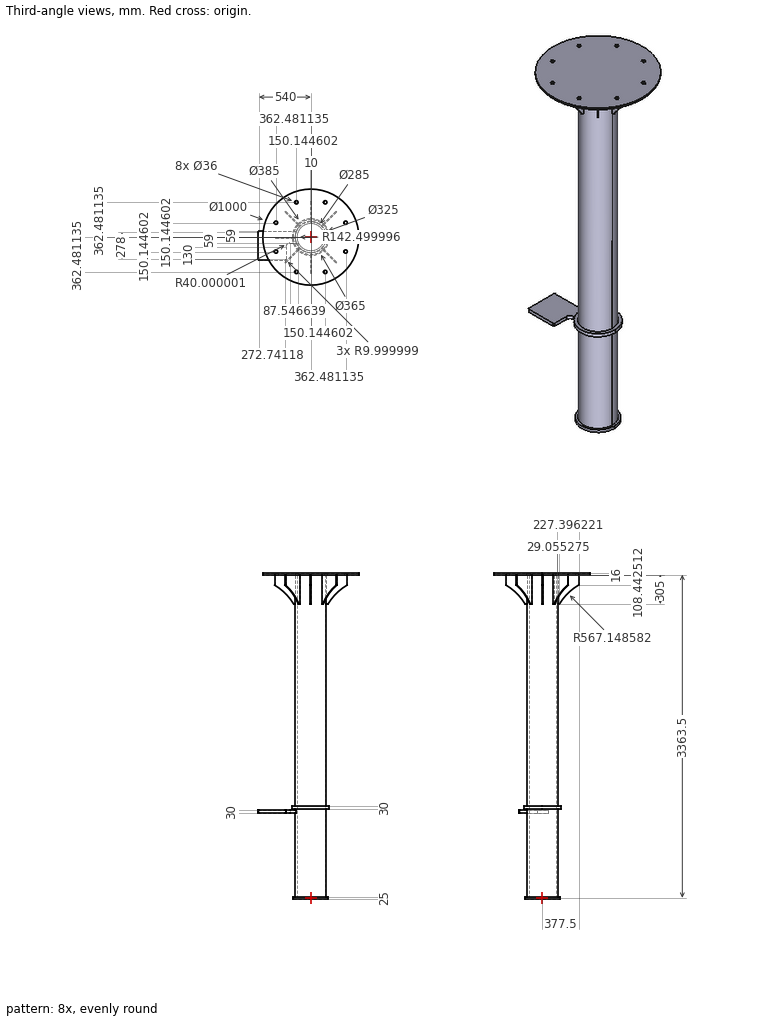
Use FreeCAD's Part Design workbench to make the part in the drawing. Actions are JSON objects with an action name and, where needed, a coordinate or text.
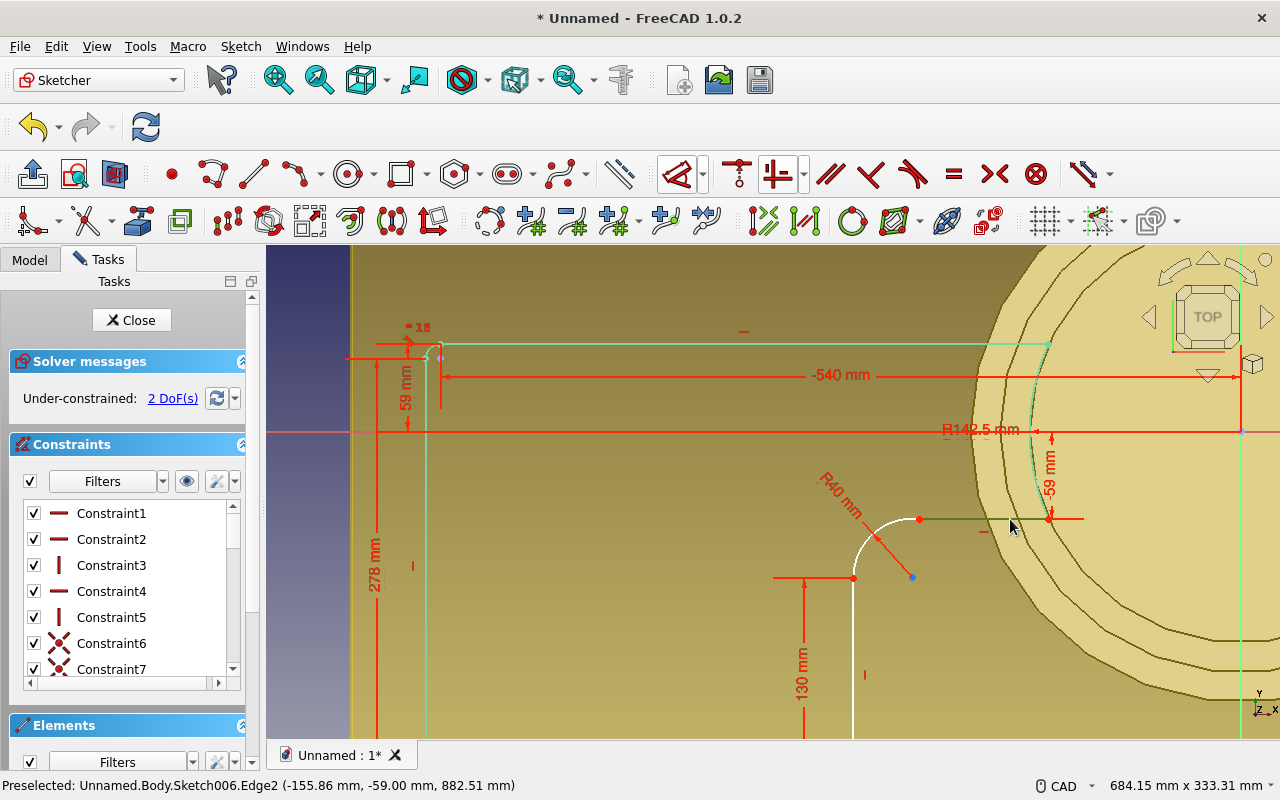
{"action": "key", "text": "l"}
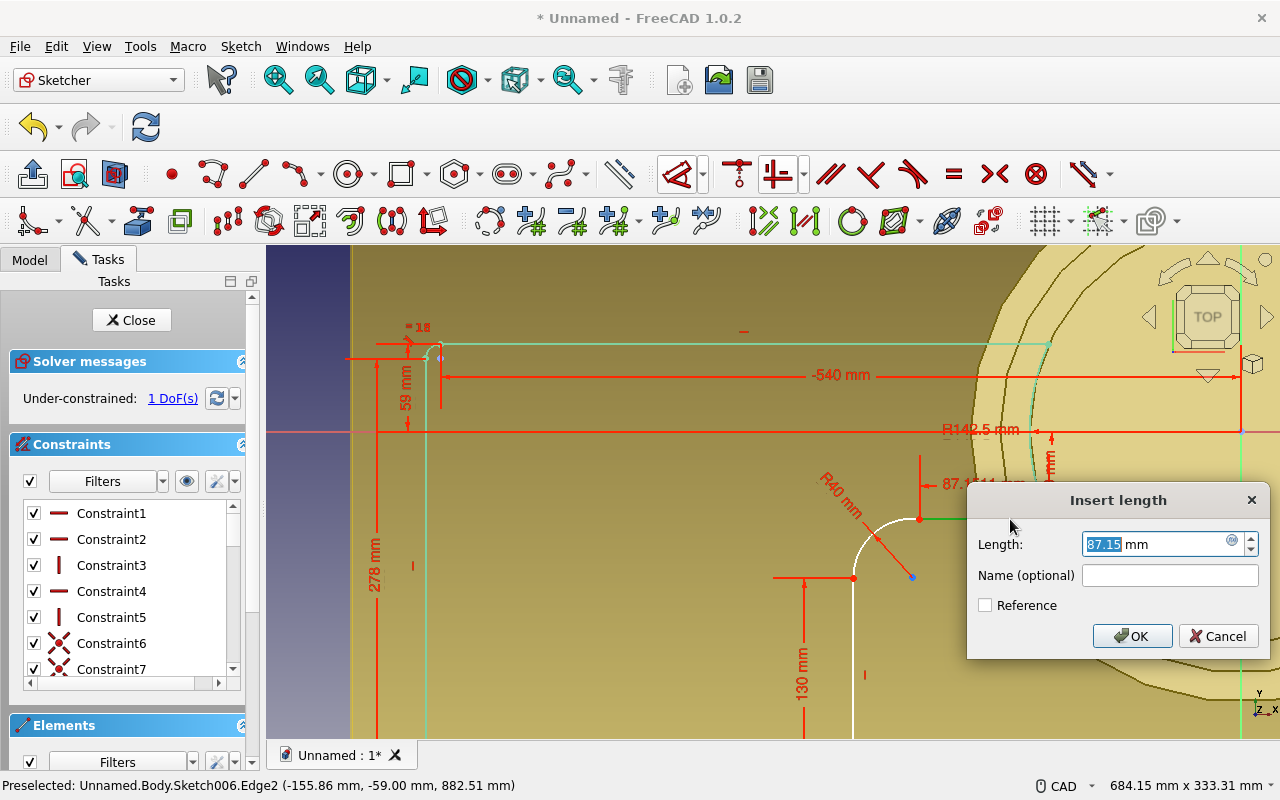
{"action": "type", "text": "87.546639"}
{"action": "key", "text": "Return"}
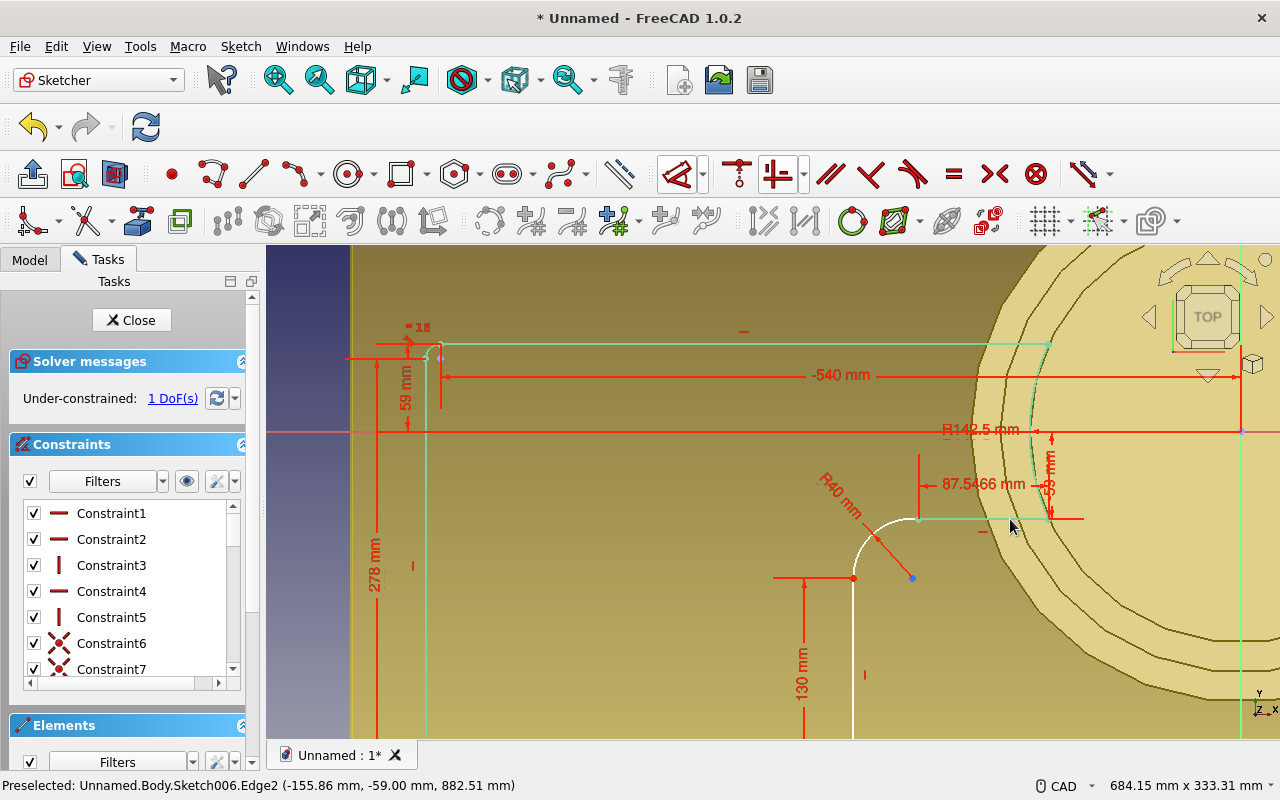
{"action": "scroll", "coordinate": [442, 344], "scroll_direction": "down", "scroll_amount": 2}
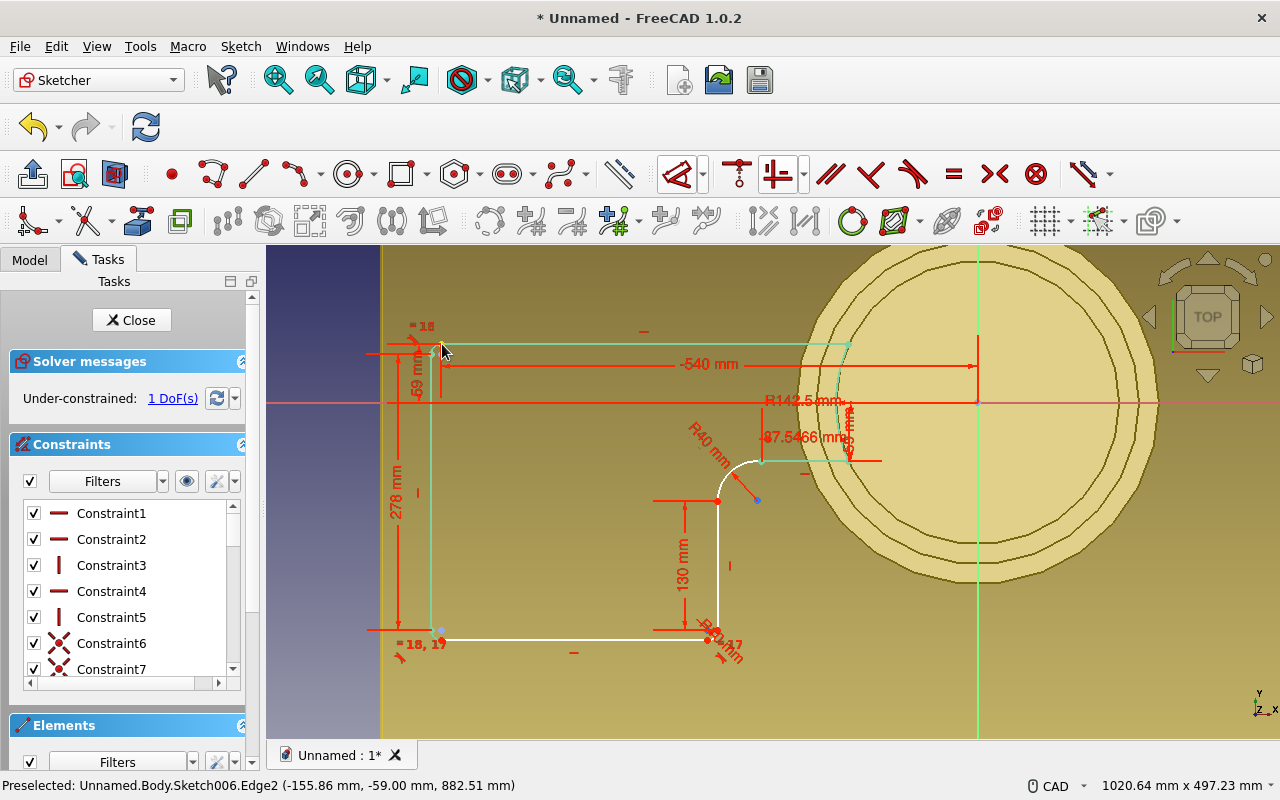
{"action": "left_click", "coordinate": [628, 640]}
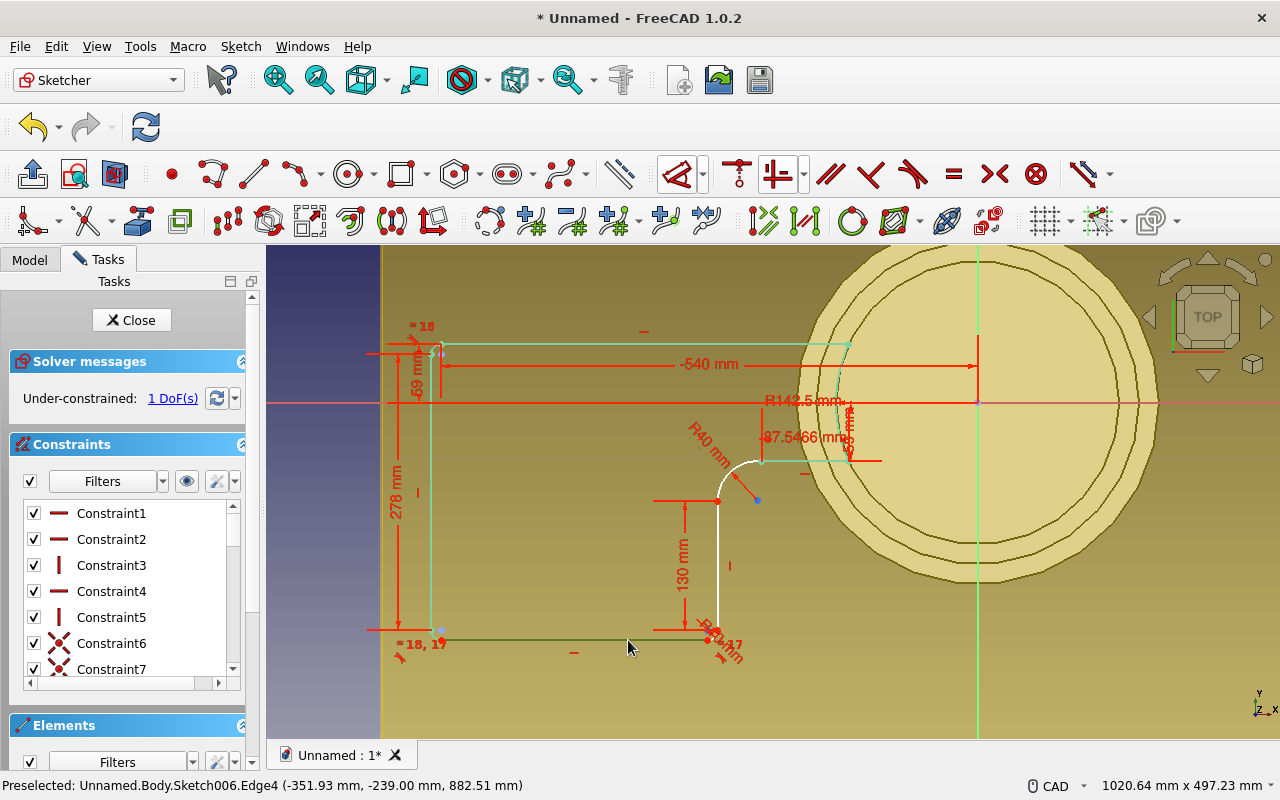
{"action": "left_click", "coordinate": [702, 174]}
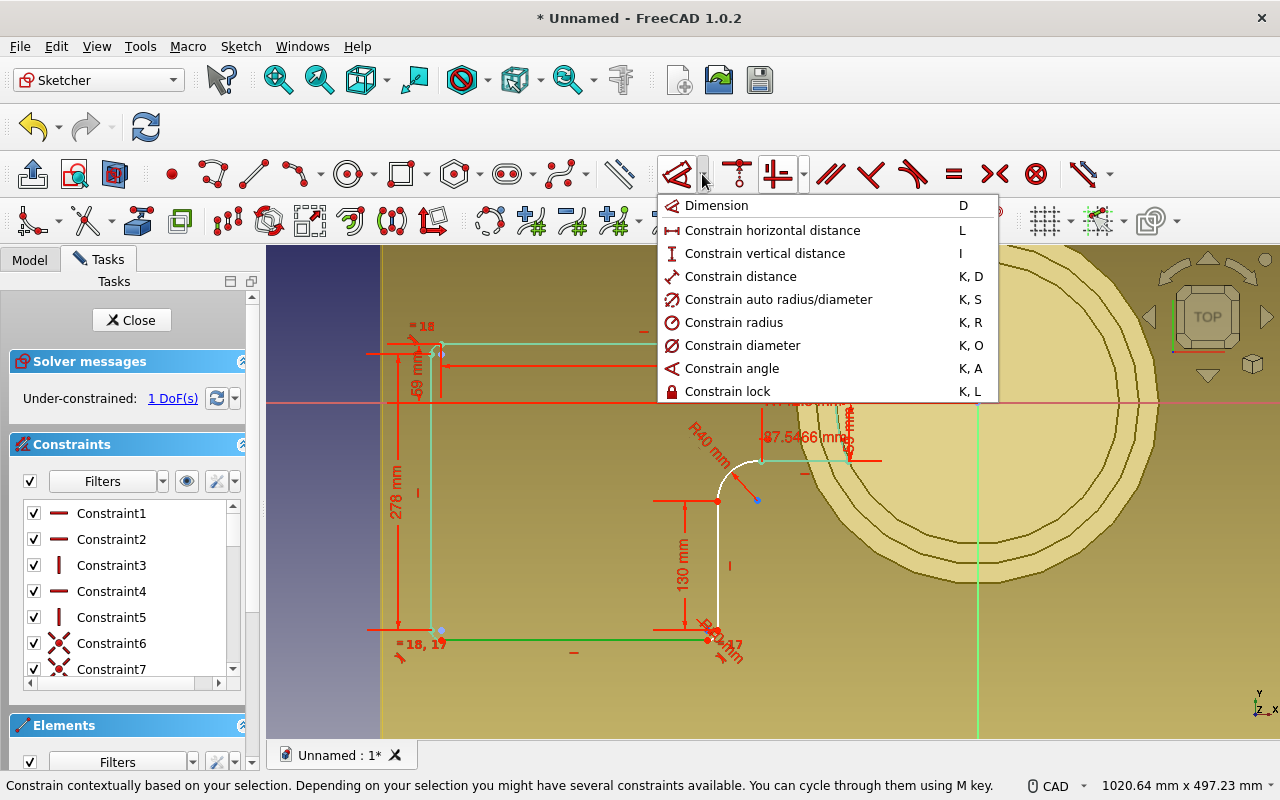
{"action": "left_click", "coordinate": [828, 230]}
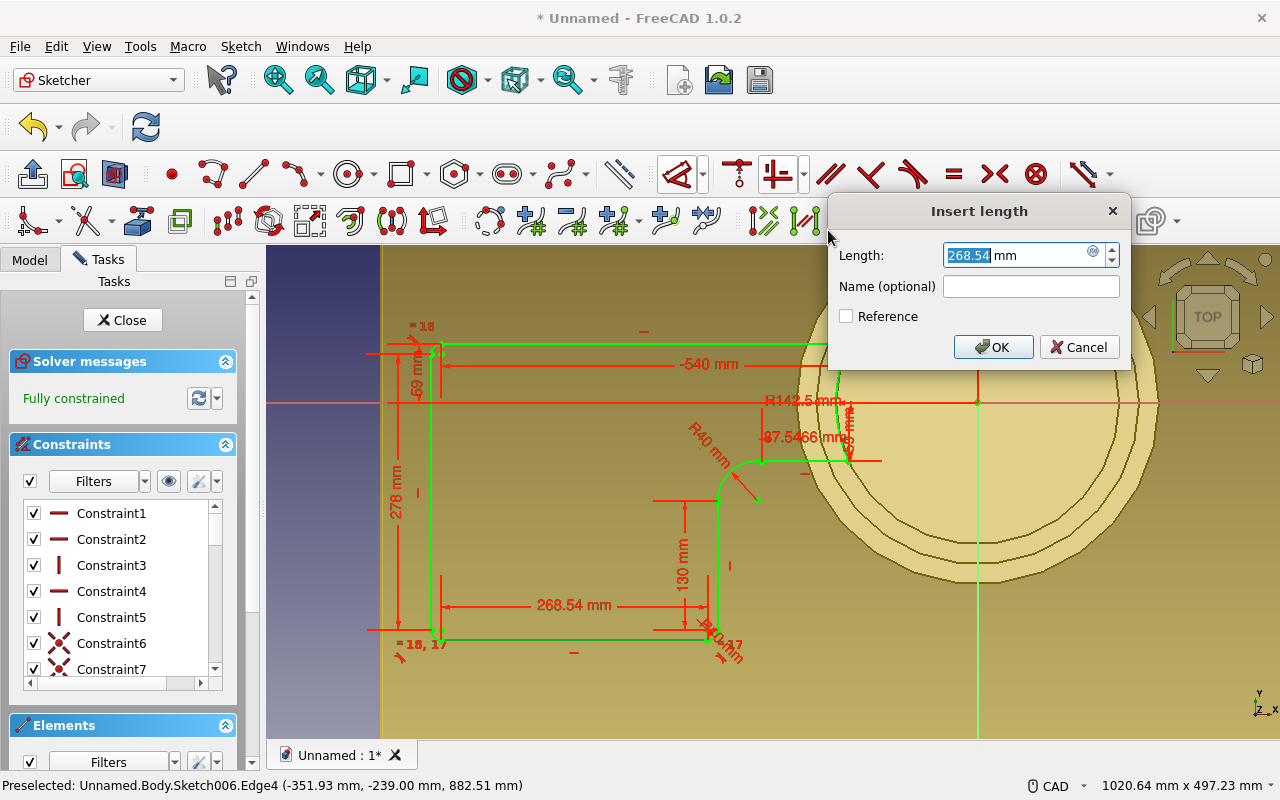
{"action": "type", "text": "272.74118"}
{"action": "key", "text": "Return"}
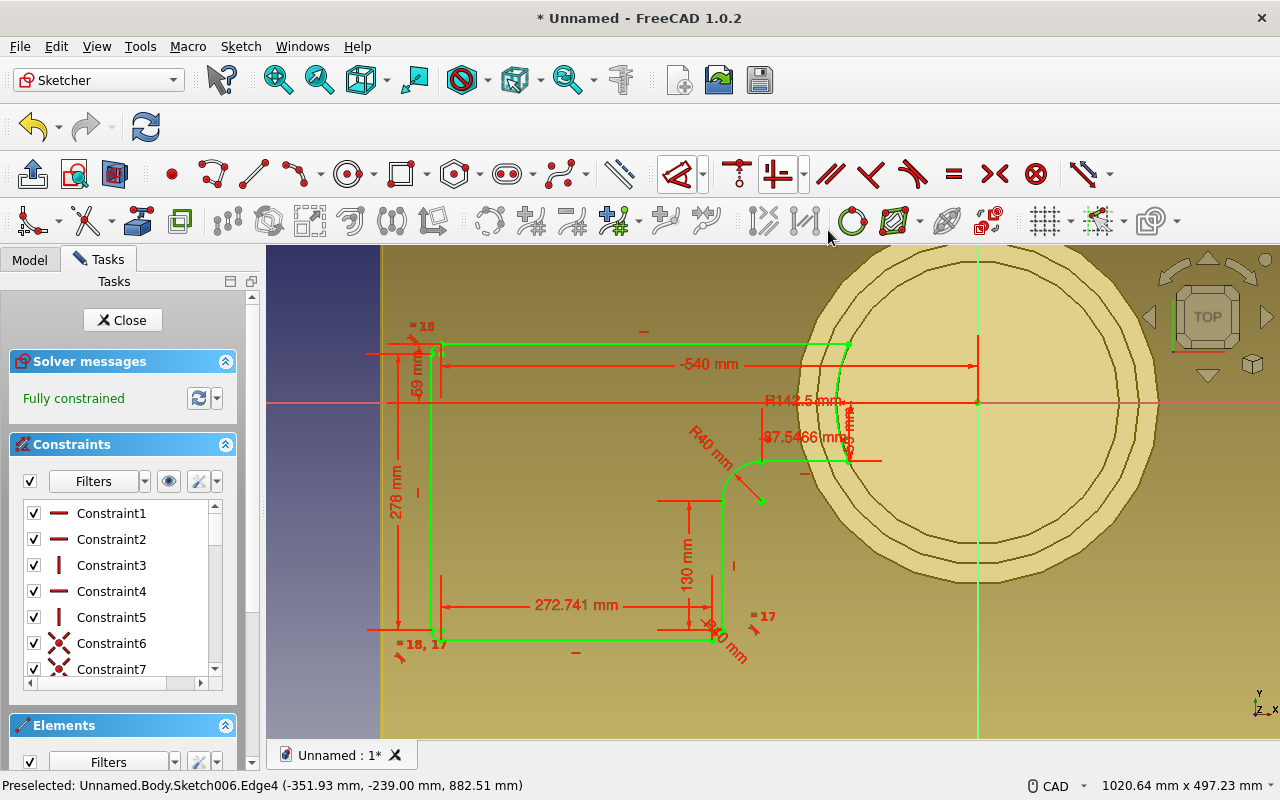
{"action": "left_click", "coordinate": [123, 320]}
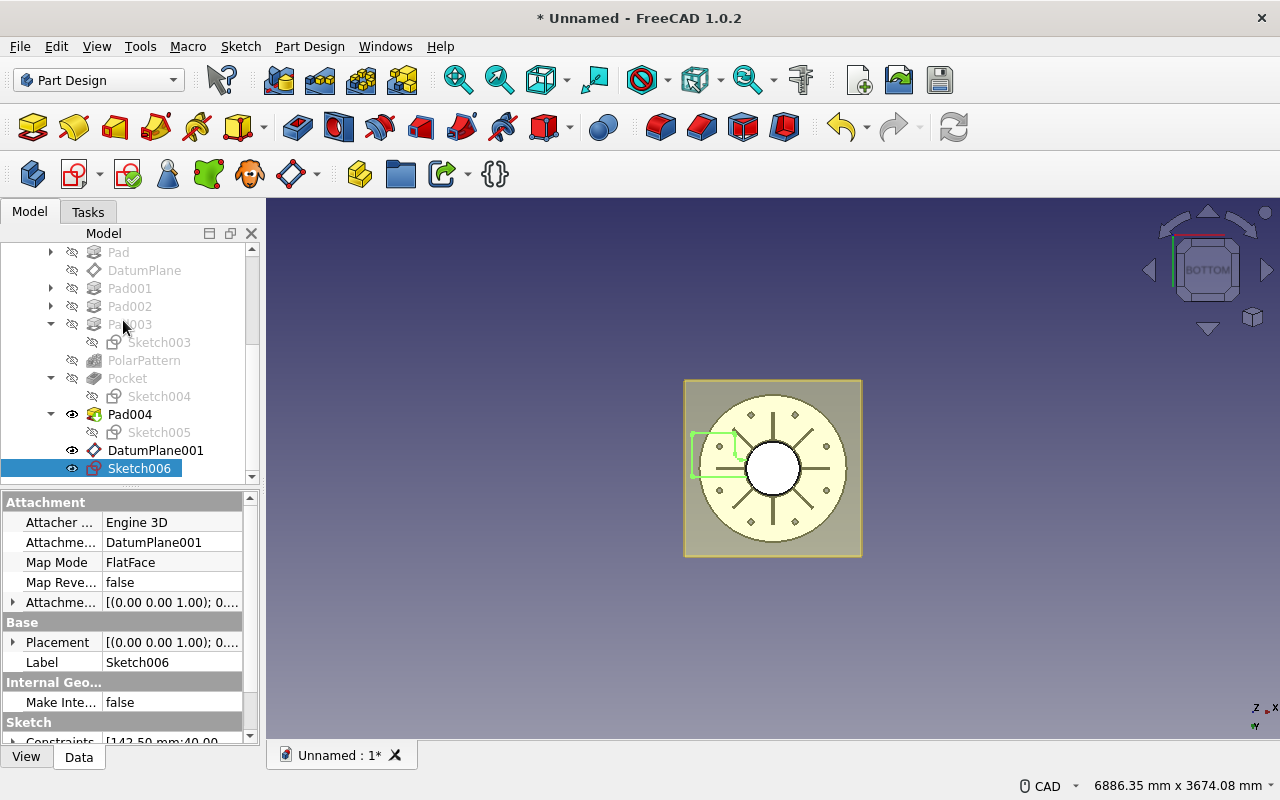
{"action": "left_click", "coordinate": [33, 128]}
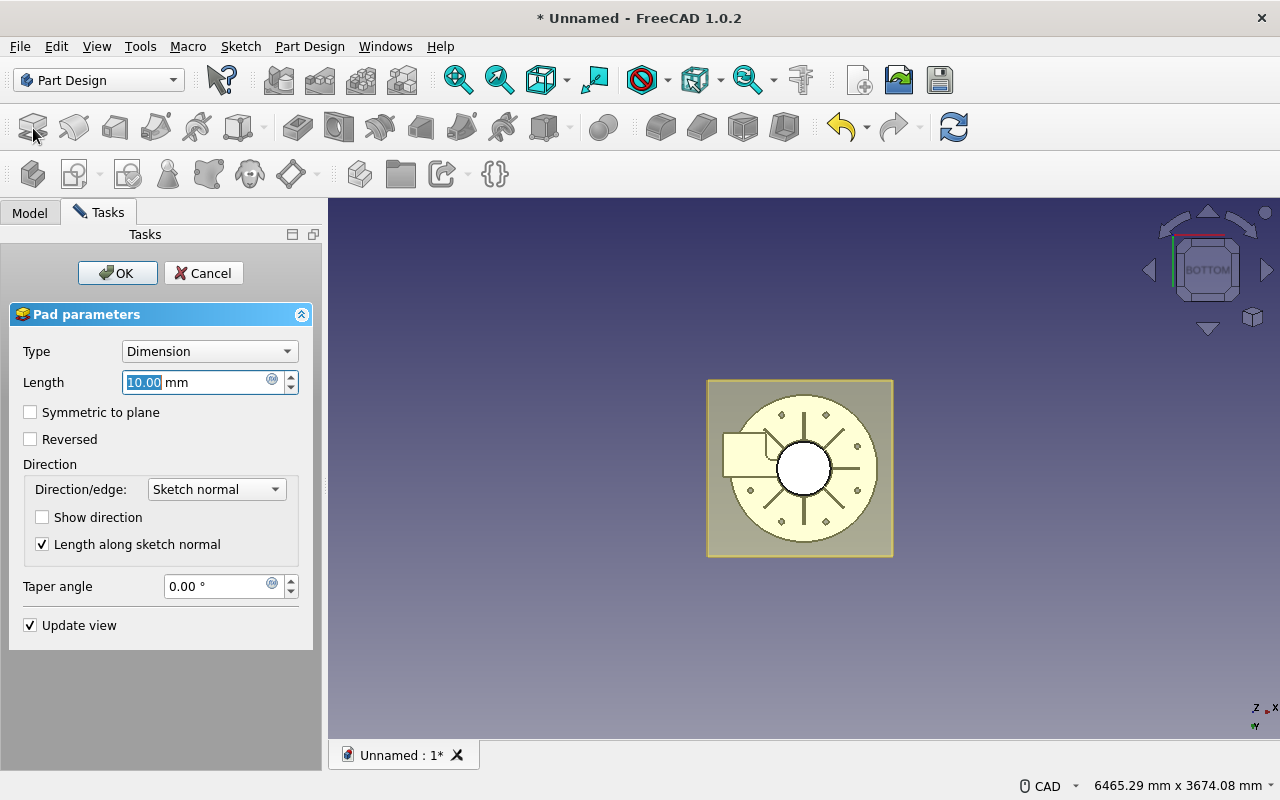
{"action": "type", "text": "30"}
{"action": "key", "text": "Tab"}